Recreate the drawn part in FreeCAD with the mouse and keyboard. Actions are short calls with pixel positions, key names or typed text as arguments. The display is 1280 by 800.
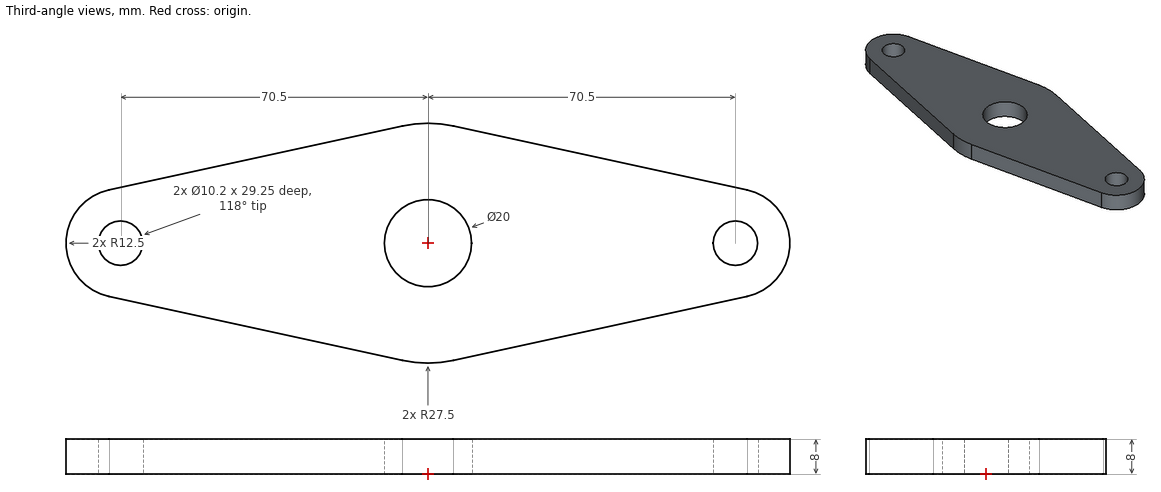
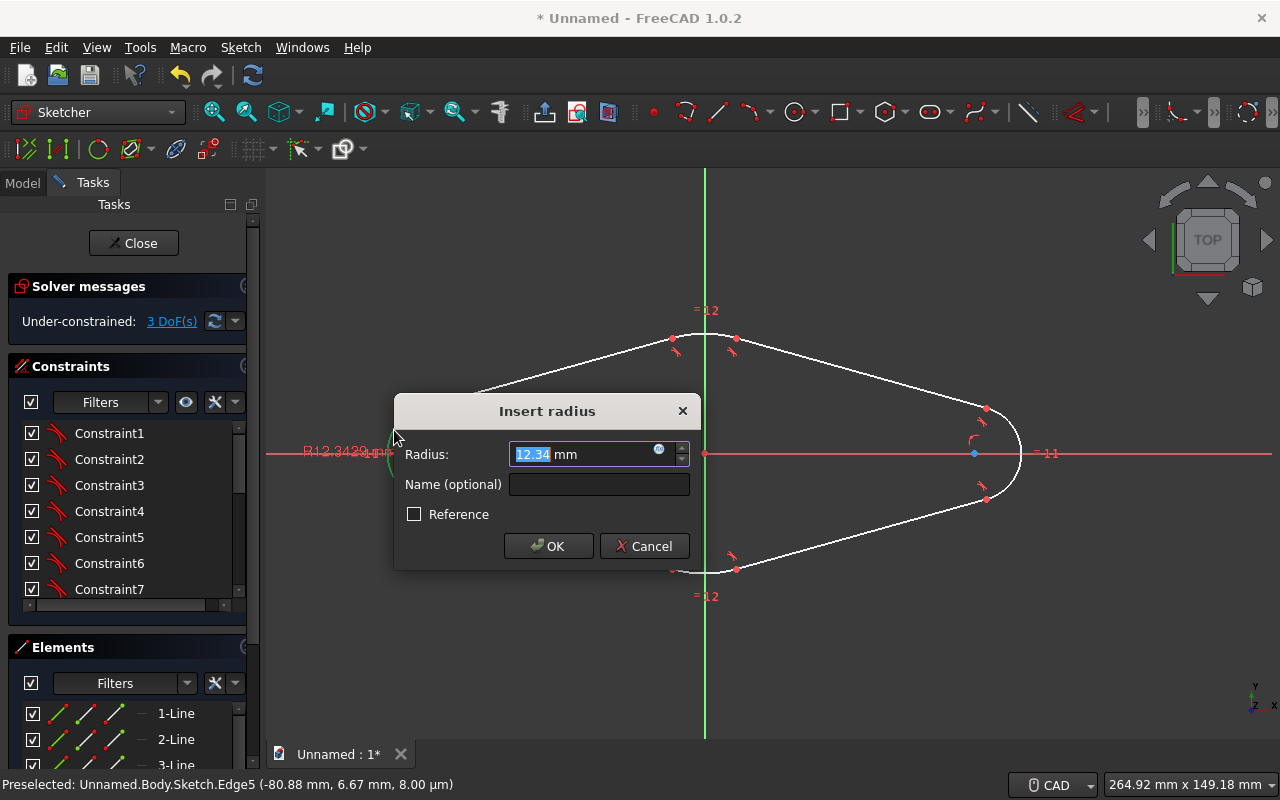
text(12.5)
key(Return)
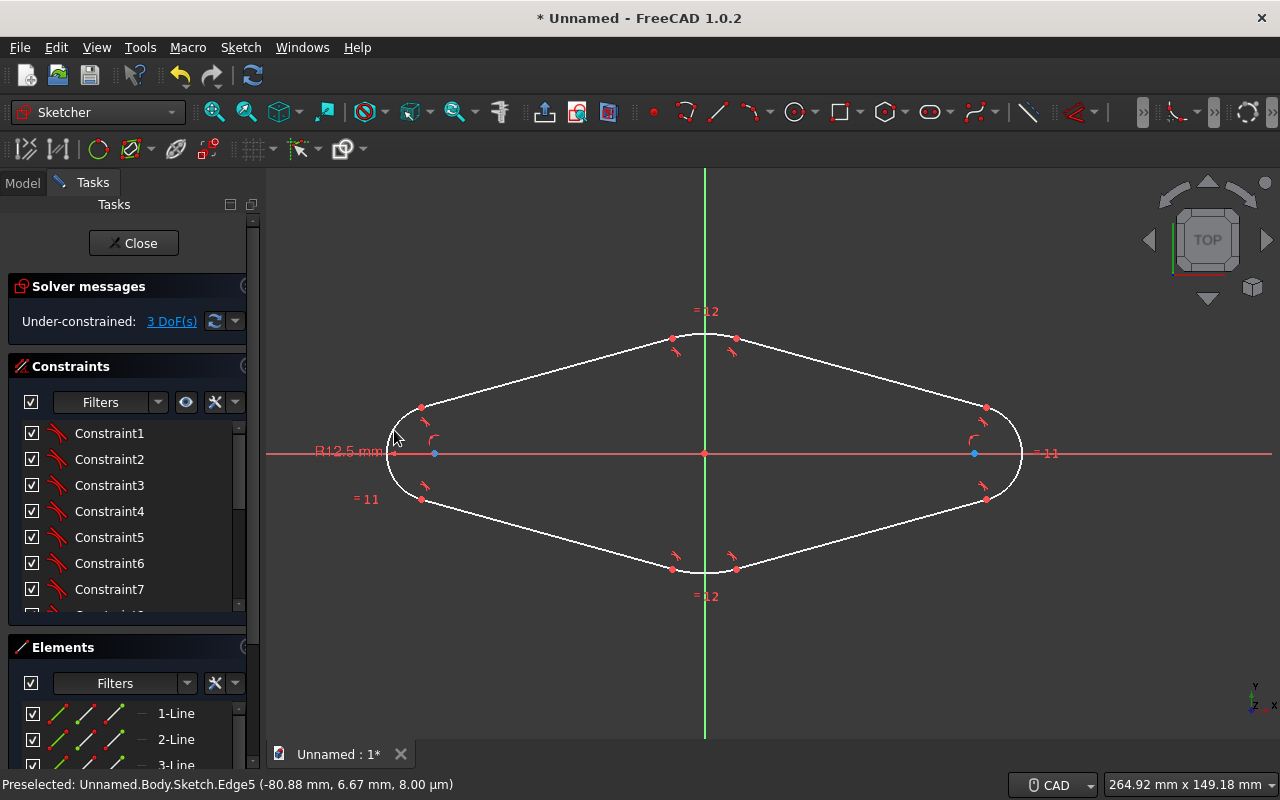
click(692, 573)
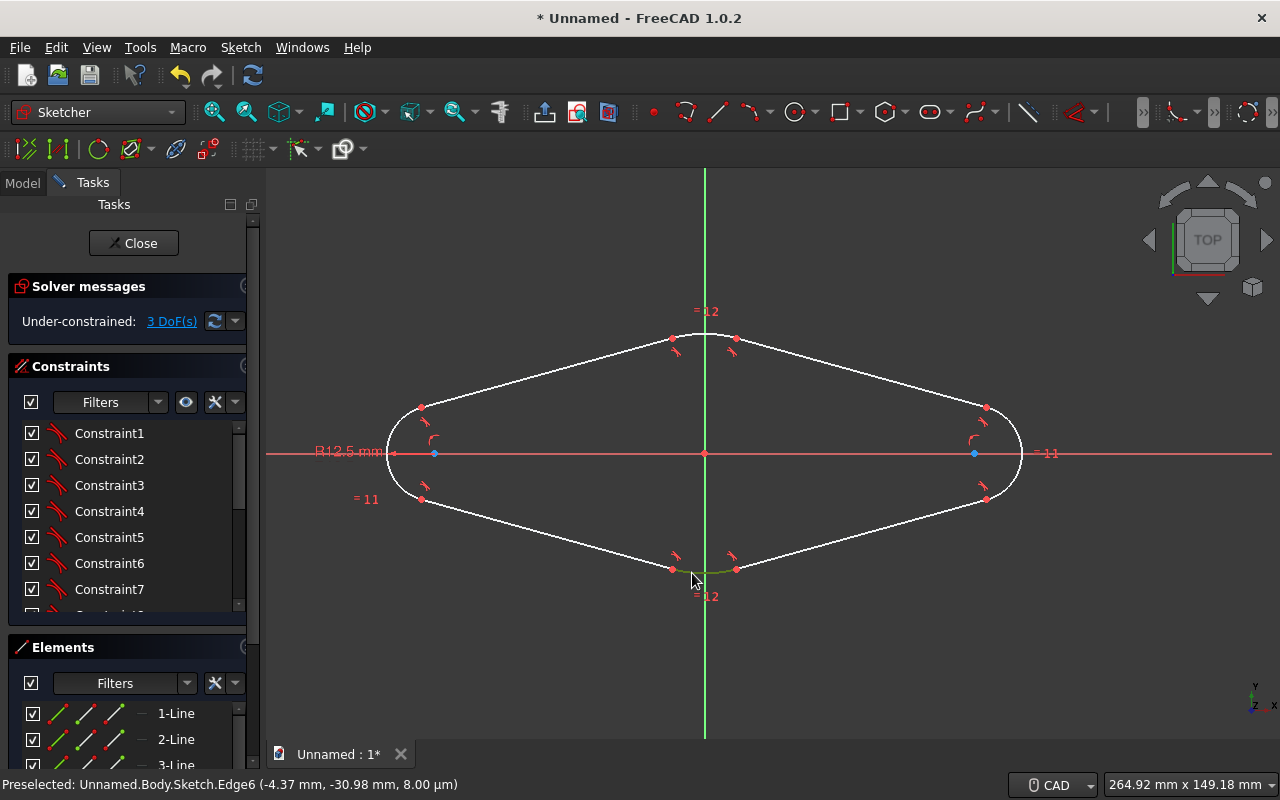
key(k)
key(r)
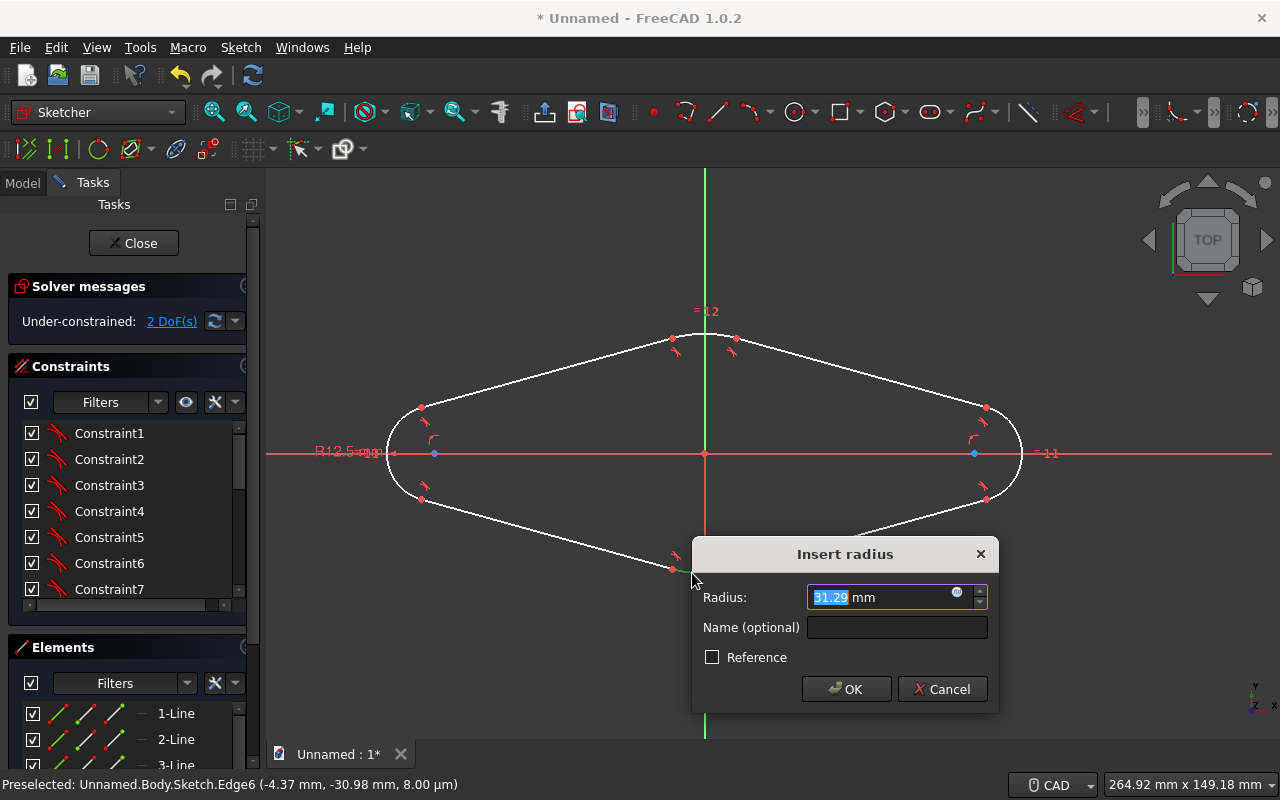
text(27.5)
key(Return)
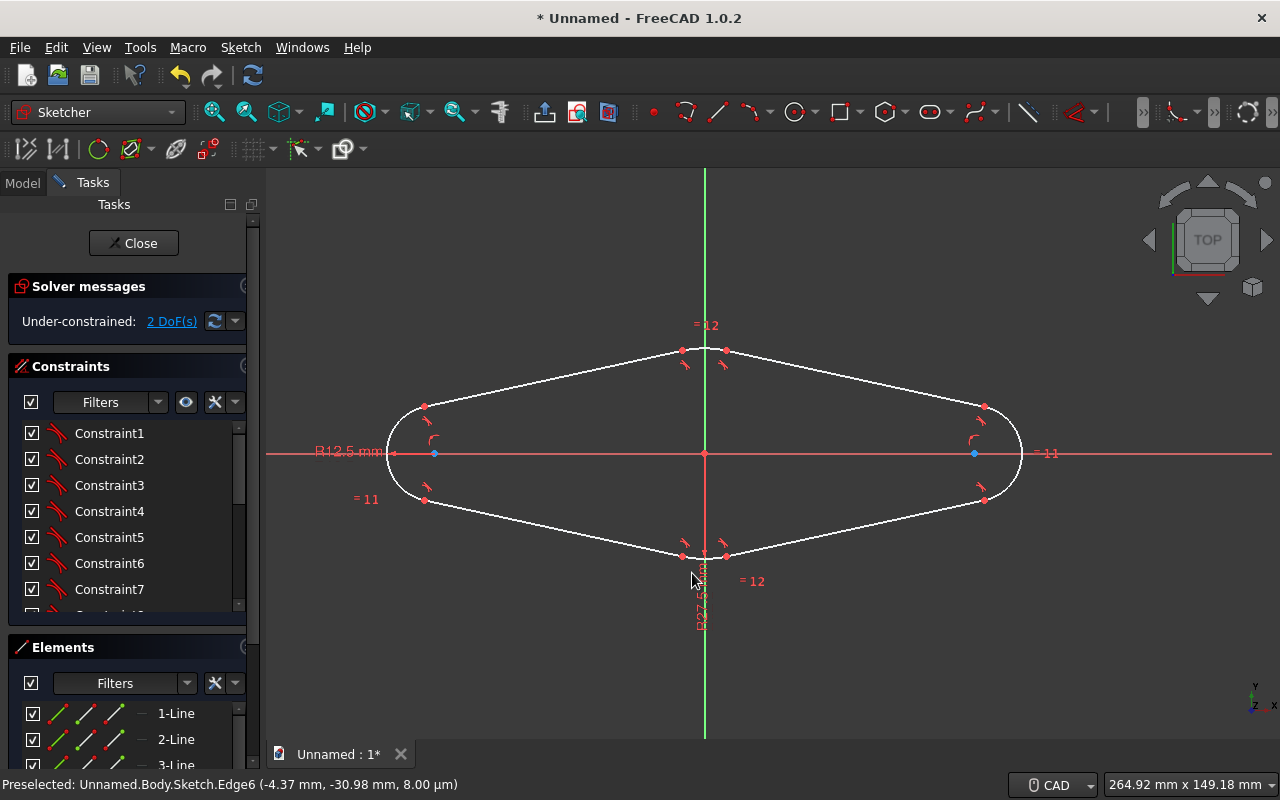
click(435, 454)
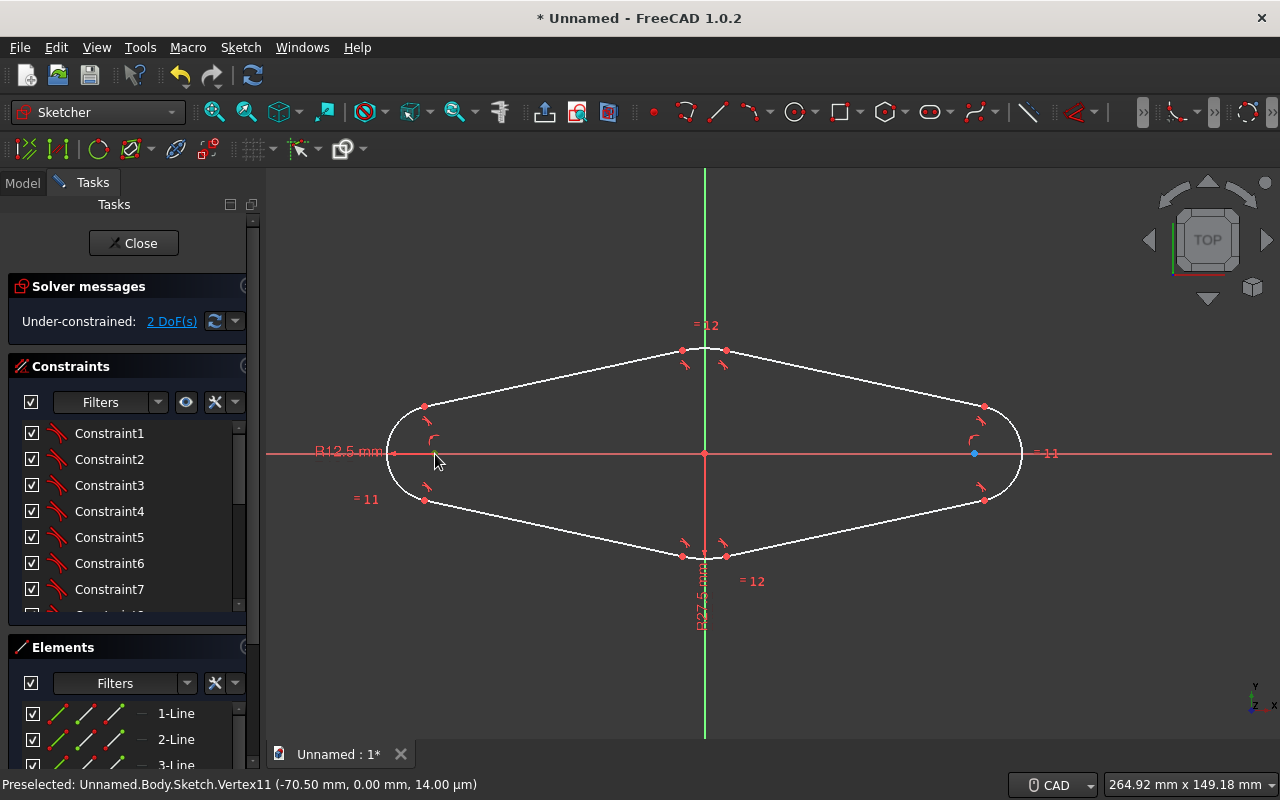
key(l)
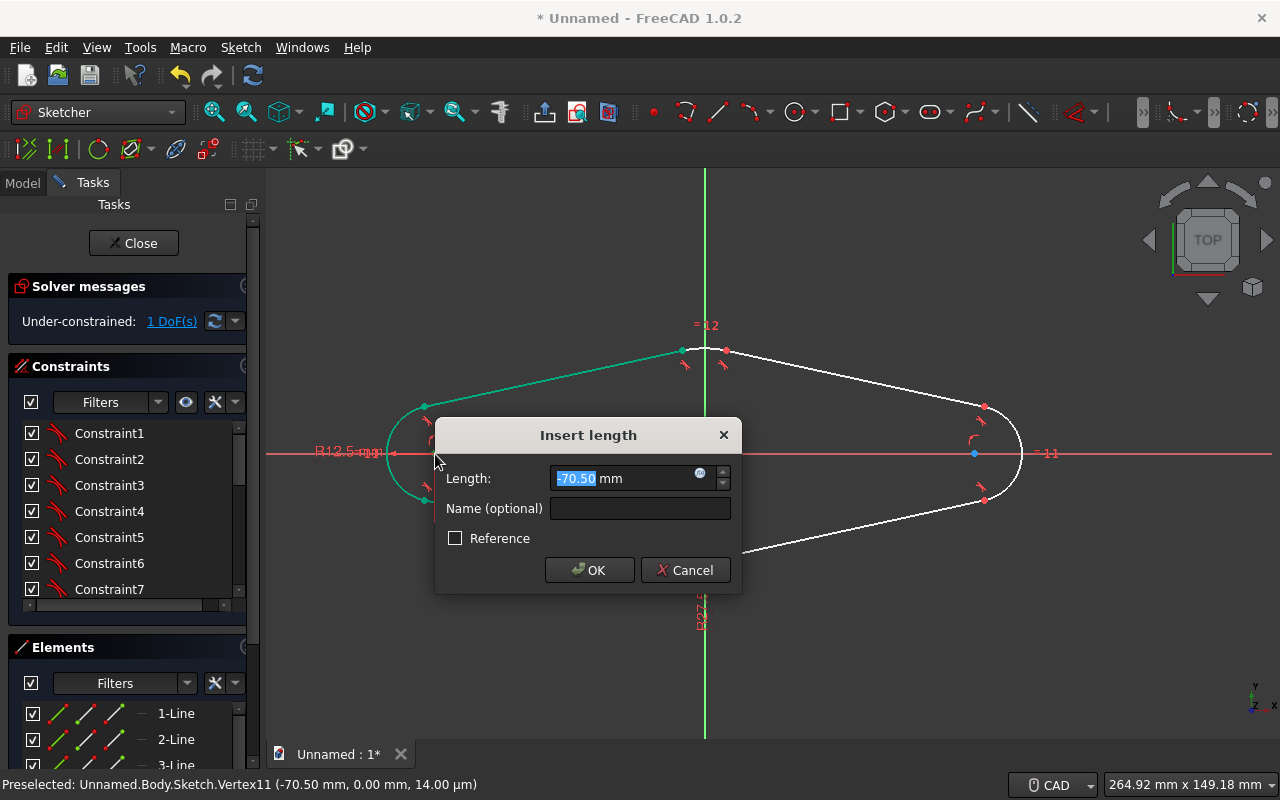
text(-70.5)
key(Return)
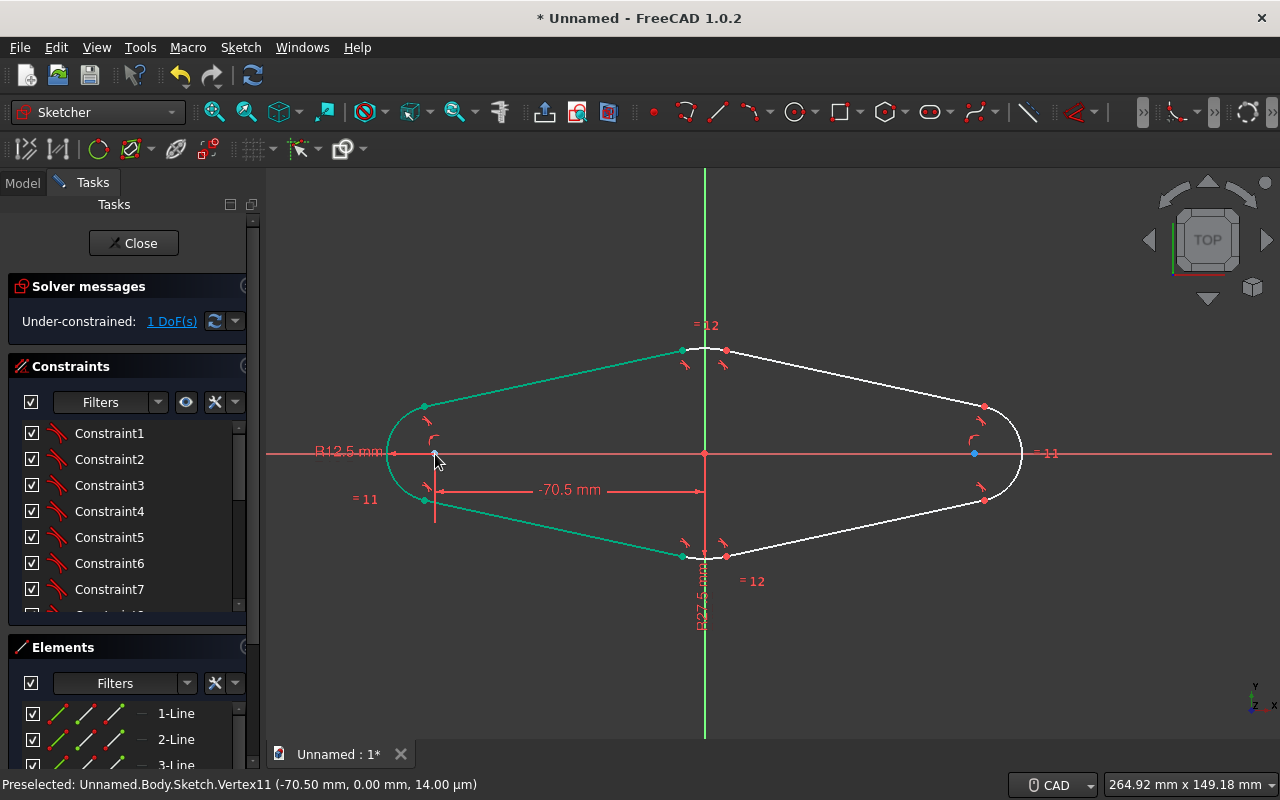
click(974, 454)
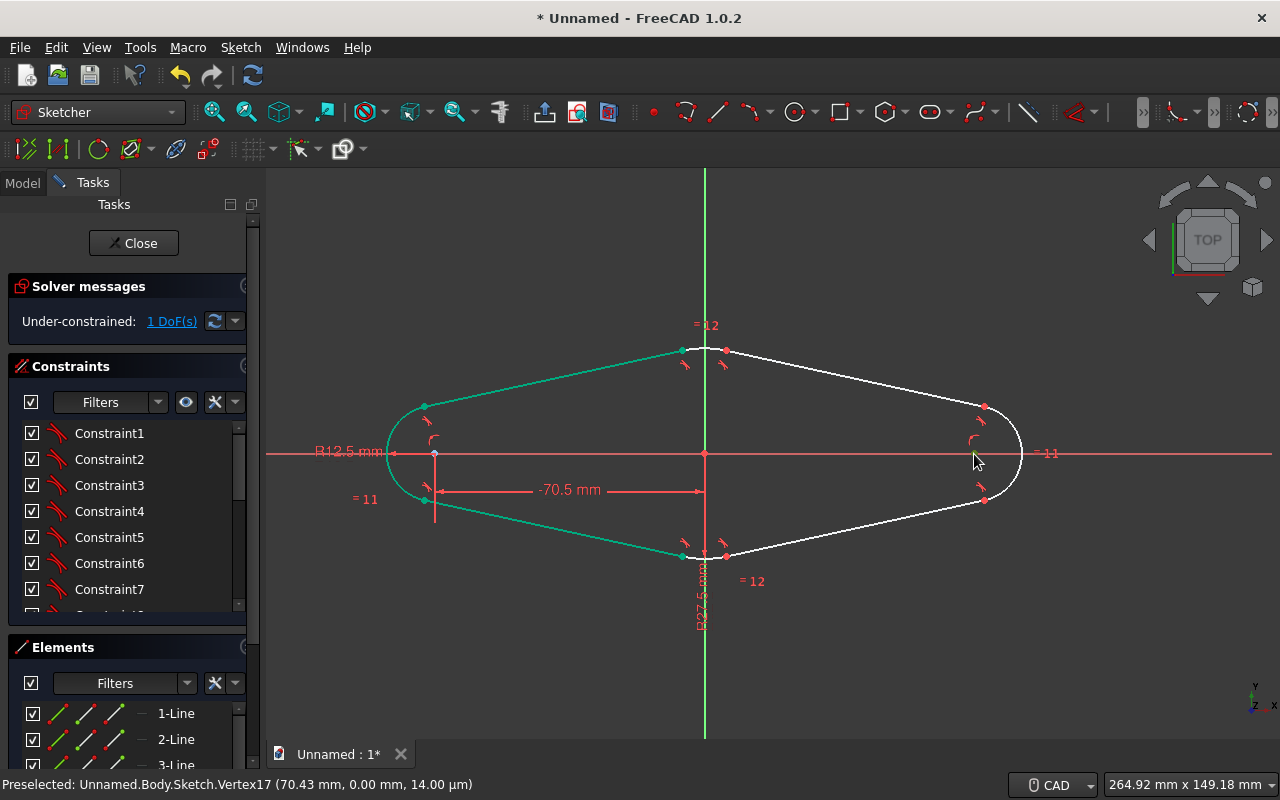
key(l)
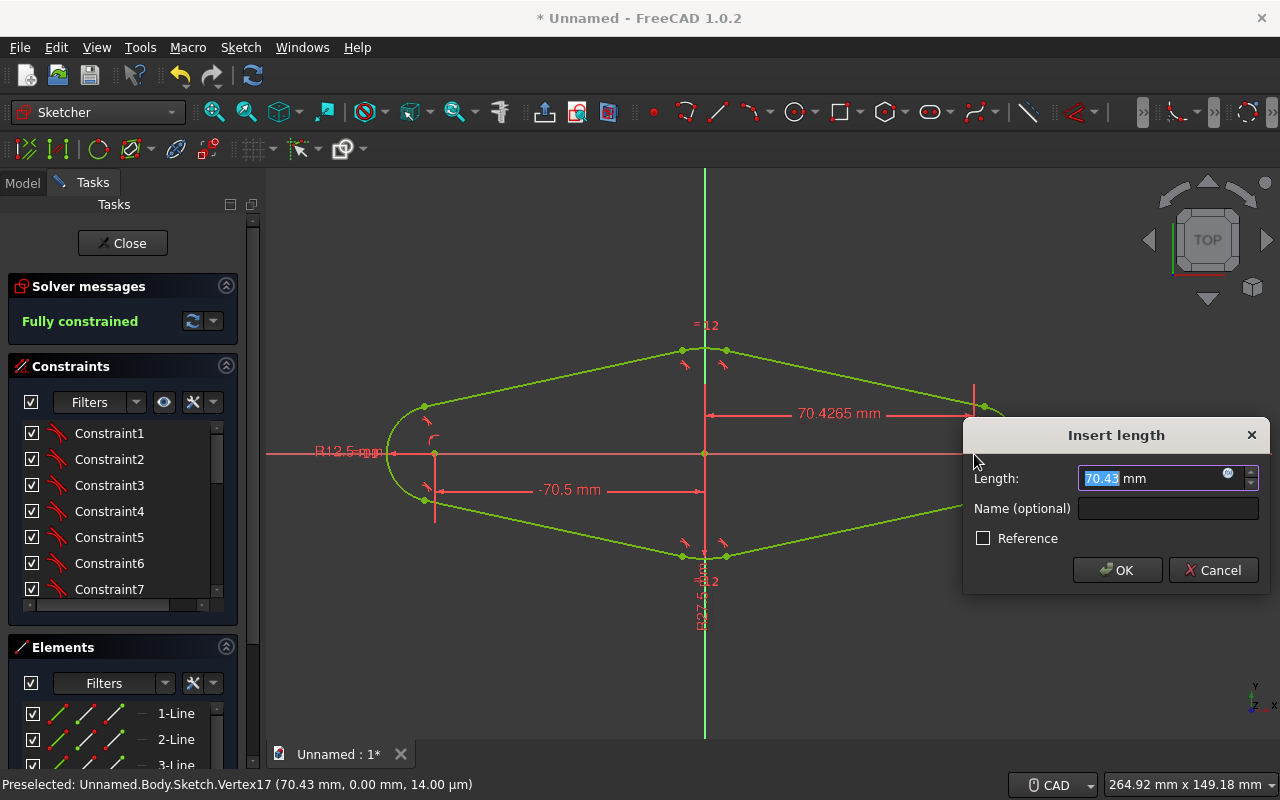
text(70.5)
key(Return)